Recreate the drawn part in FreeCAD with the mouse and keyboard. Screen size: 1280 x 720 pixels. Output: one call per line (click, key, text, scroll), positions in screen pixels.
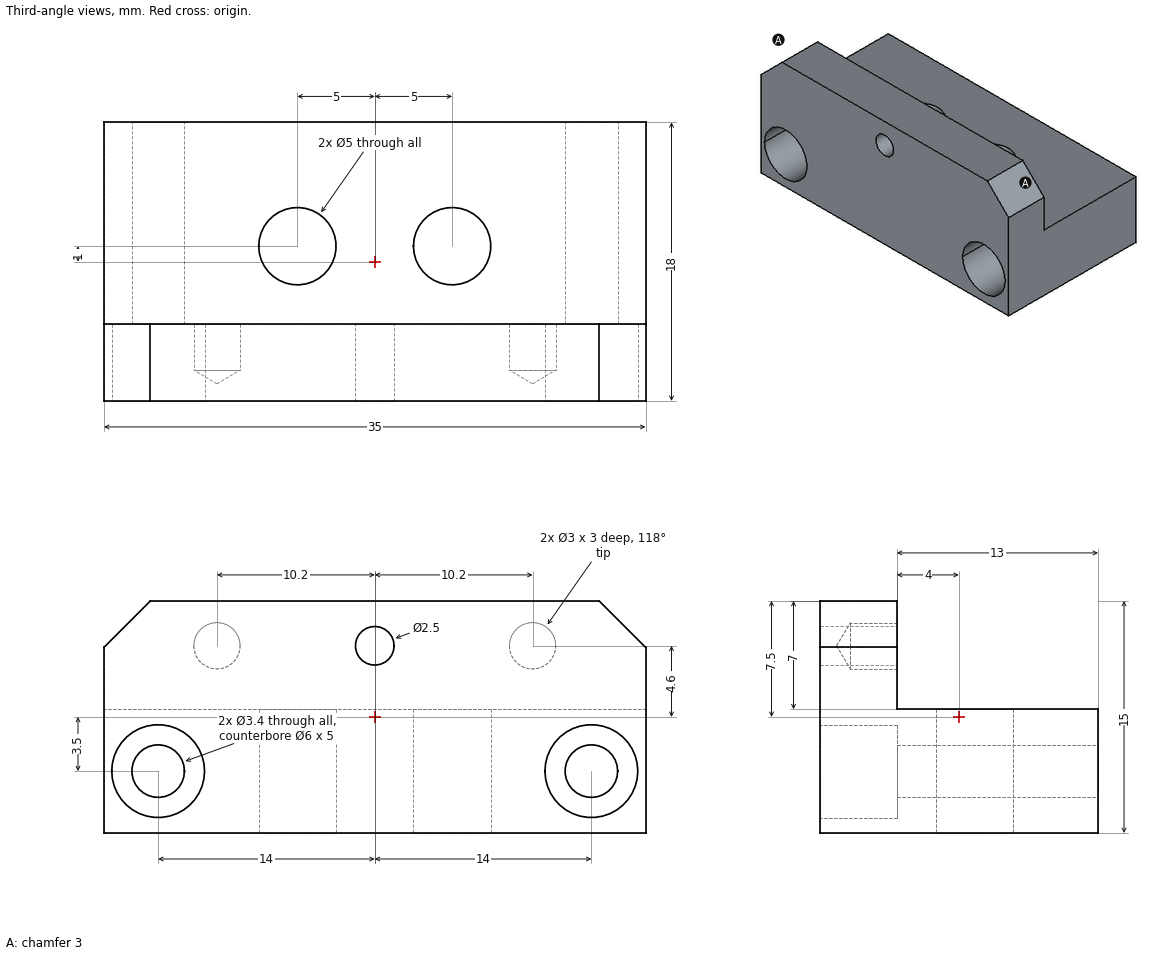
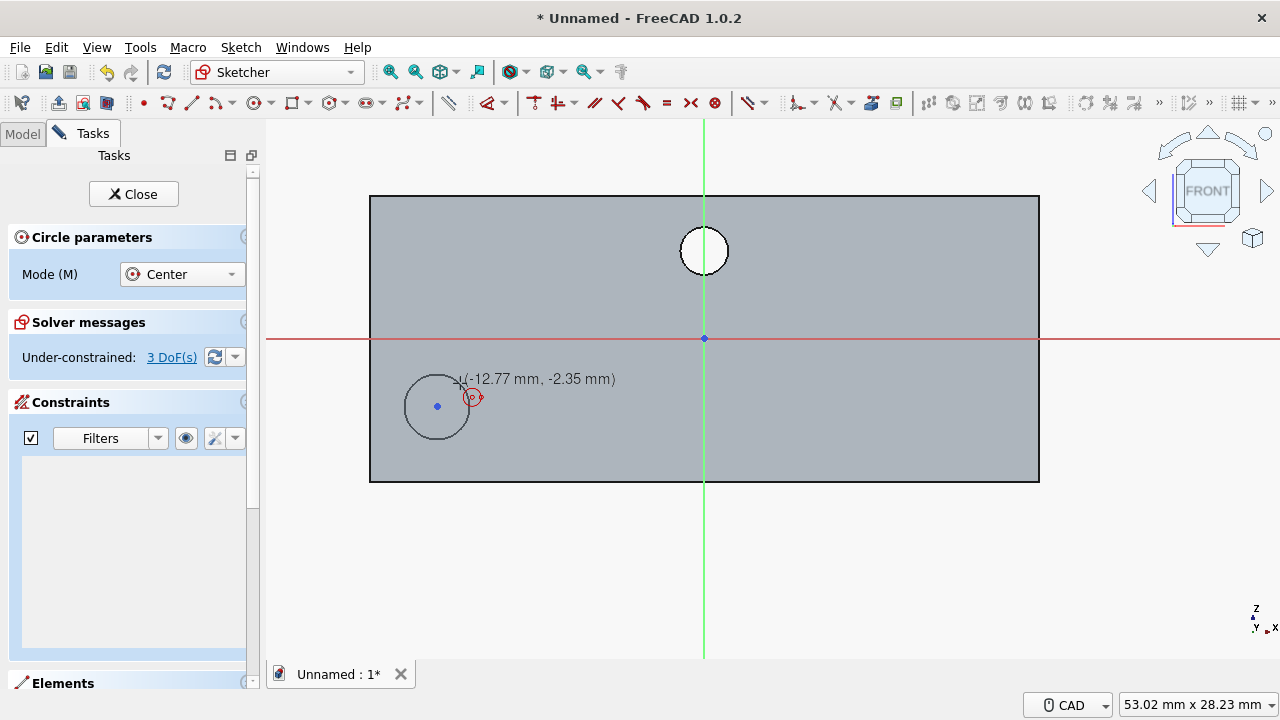
click(972, 406)
click(995, 383)
key(Escape)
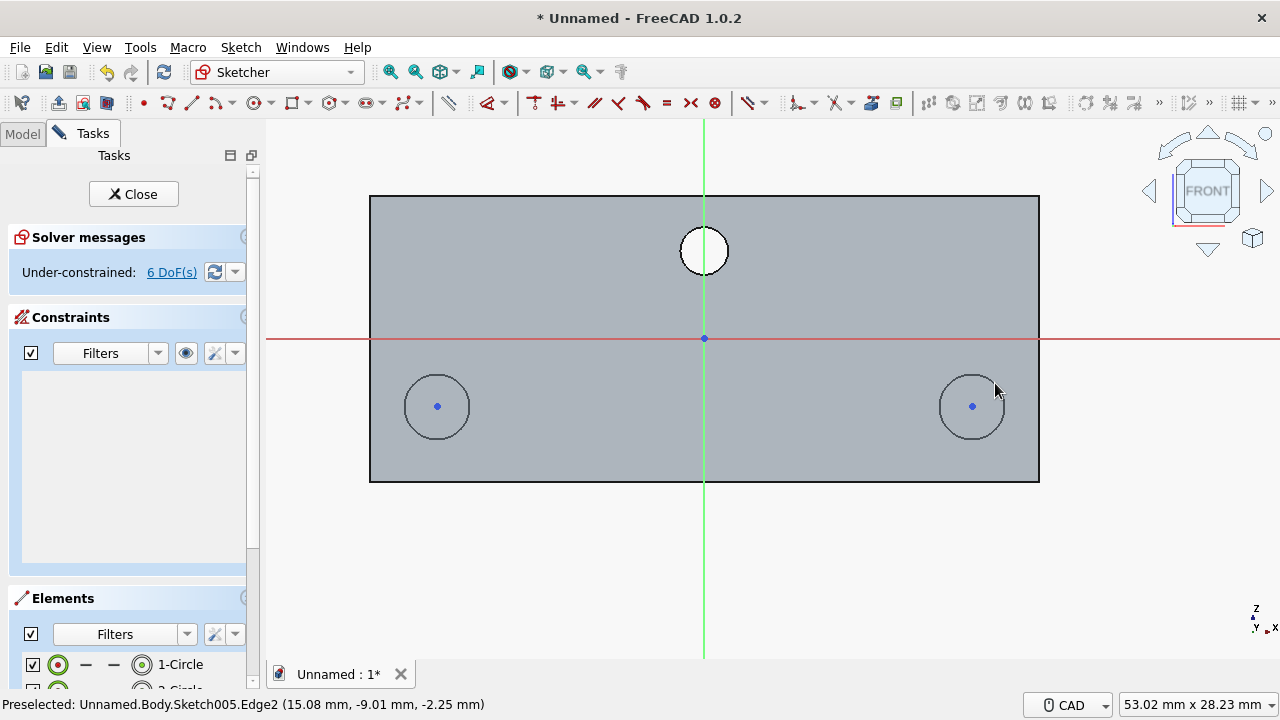
click(460, 384)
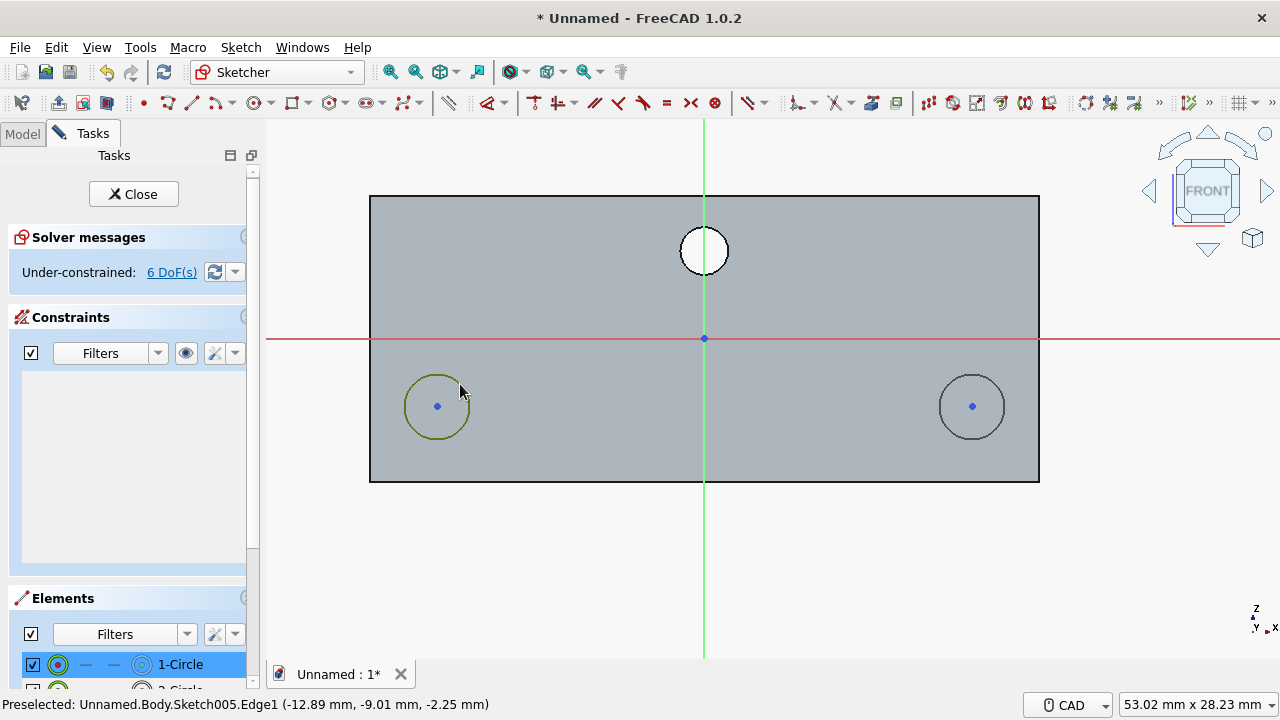
click(995, 384)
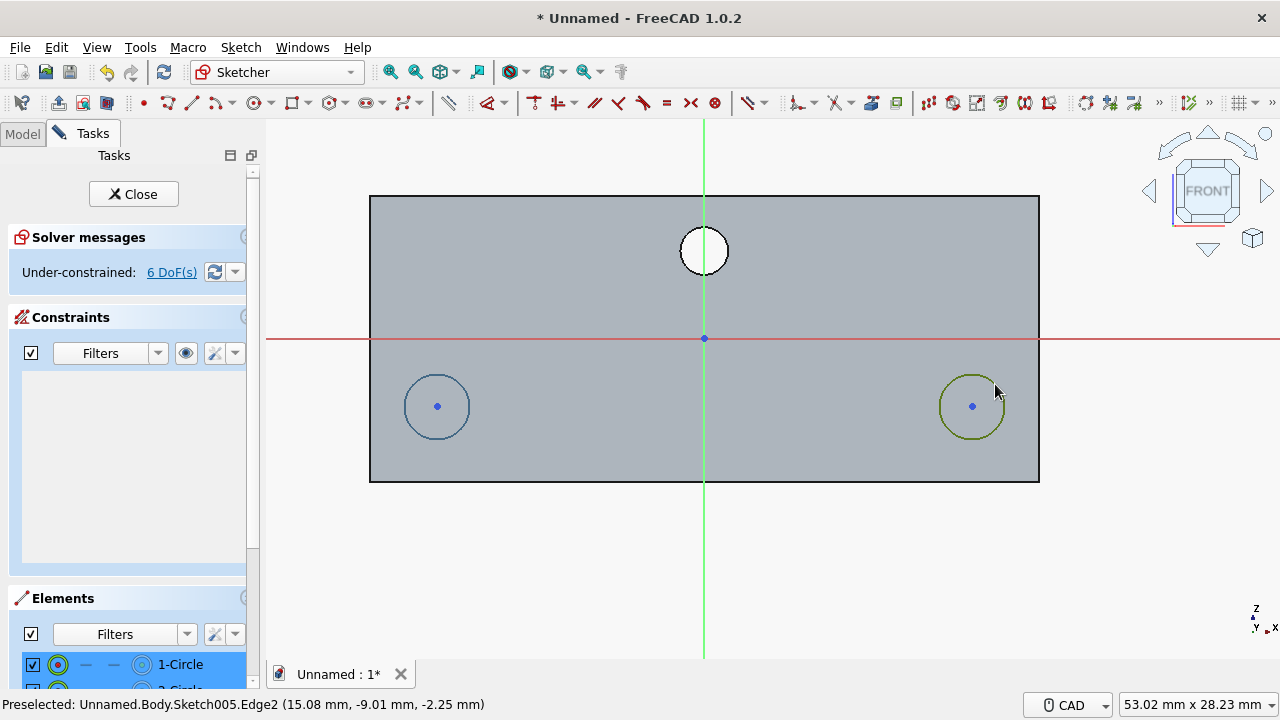
key(e)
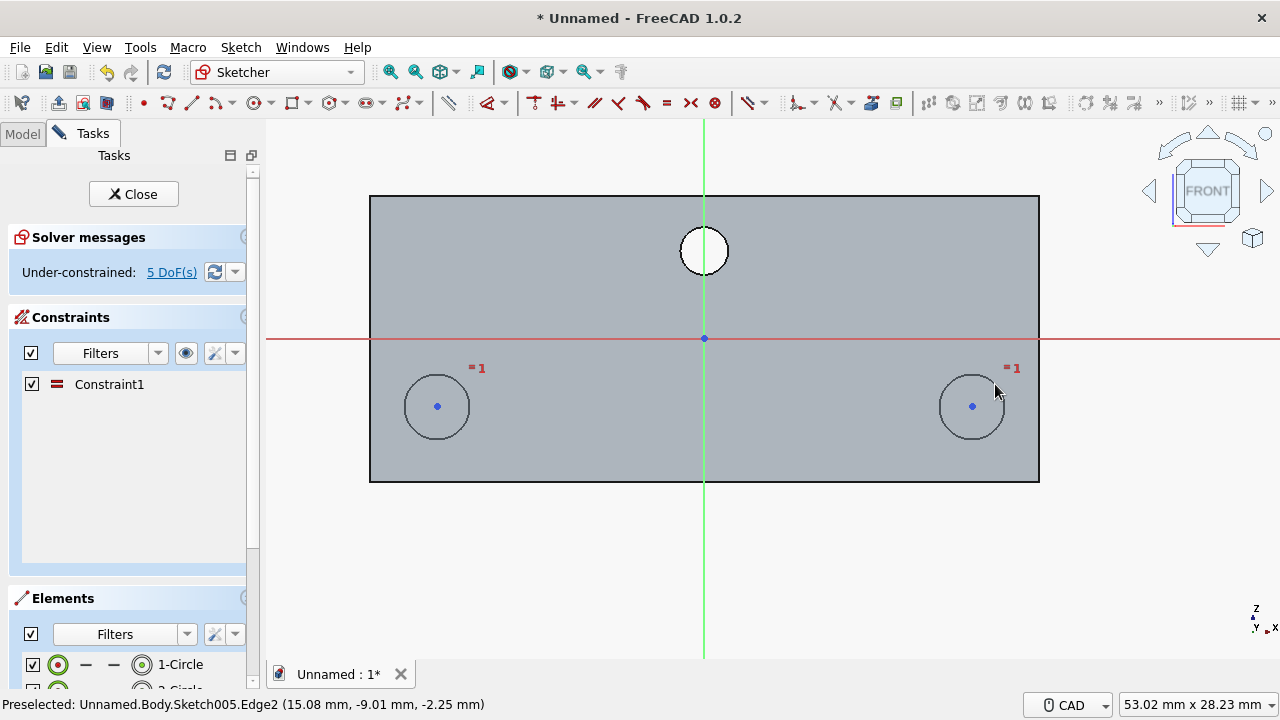
click(437, 407)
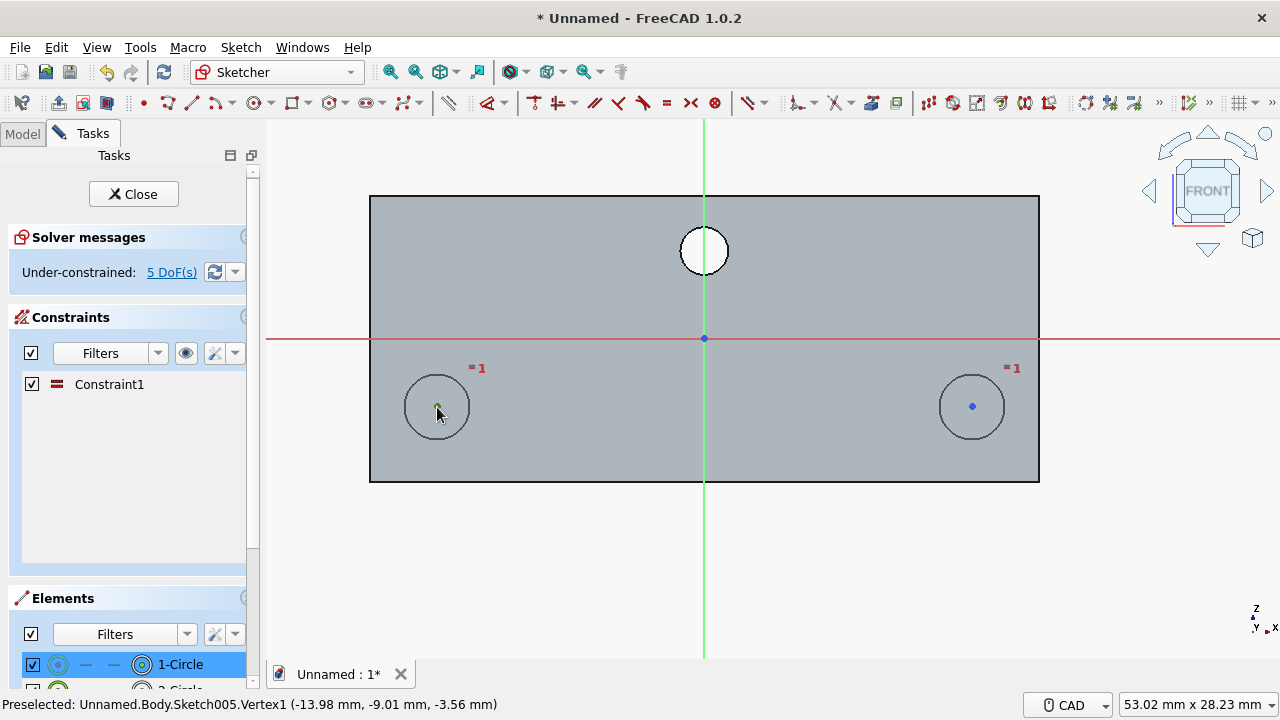
click(972, 407)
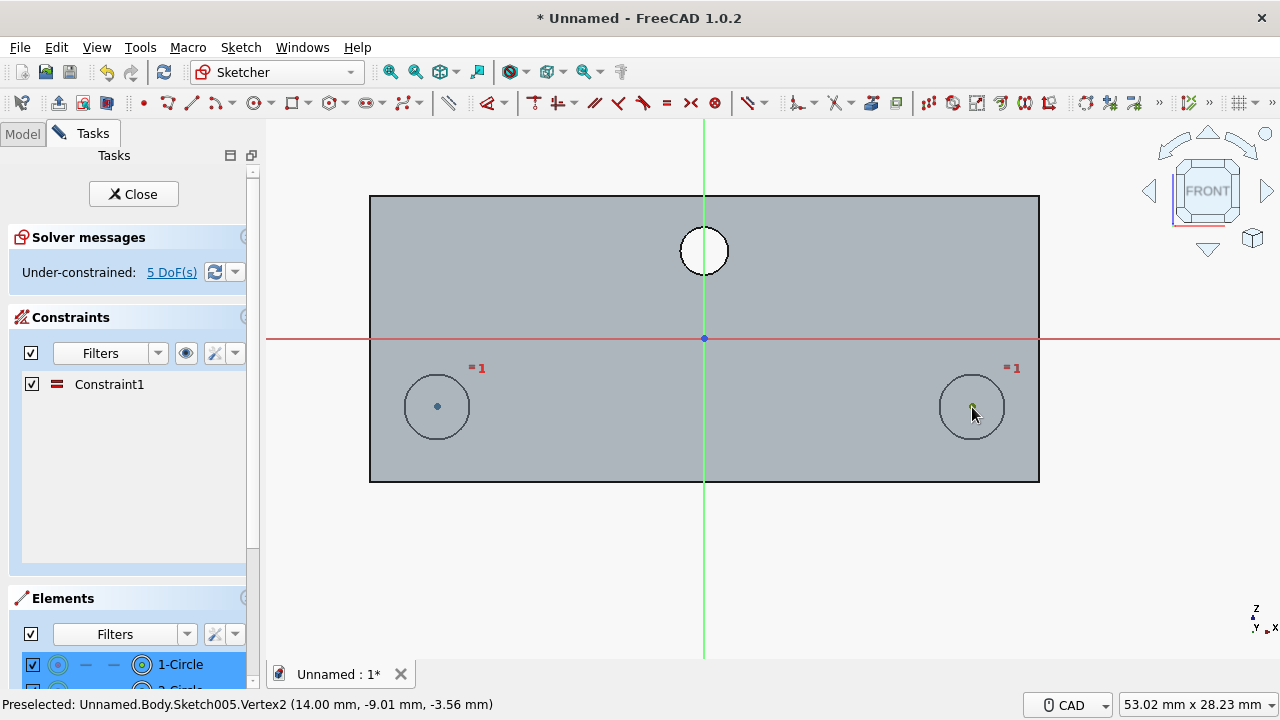
key(h)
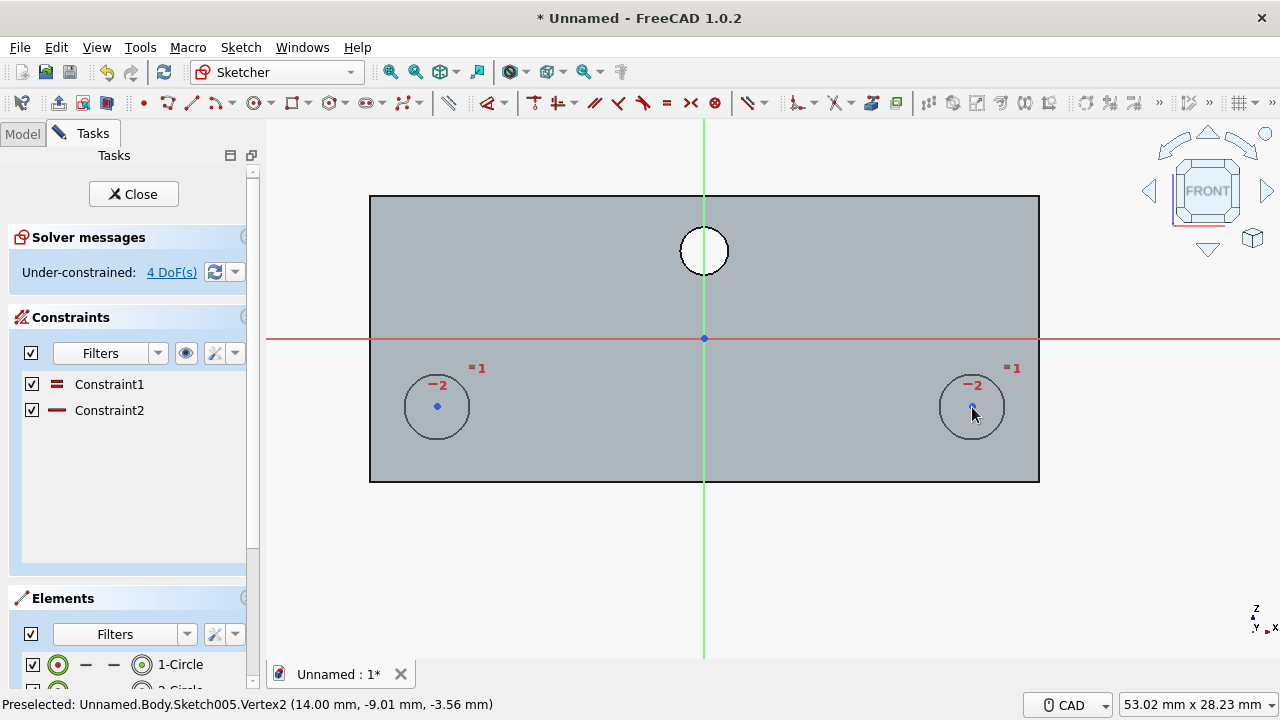
key(d)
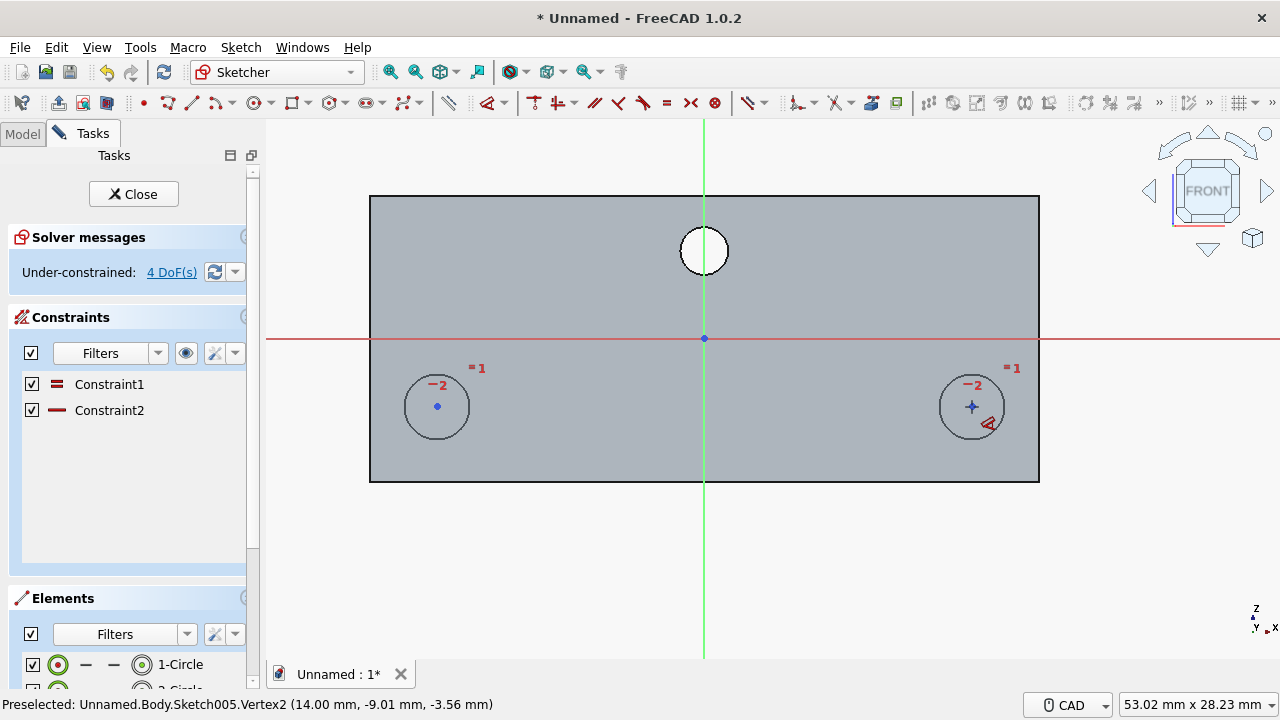
click(460, 384)
click(483, 361)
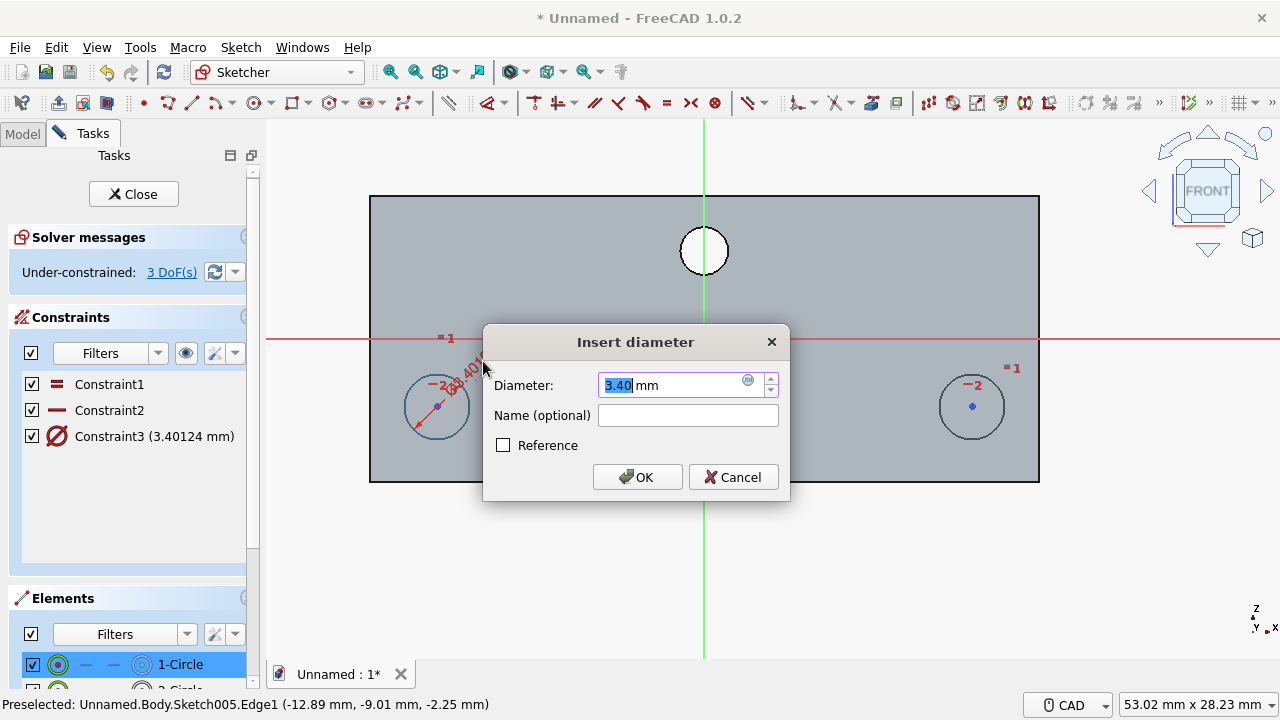
text(3.4)
key(Return)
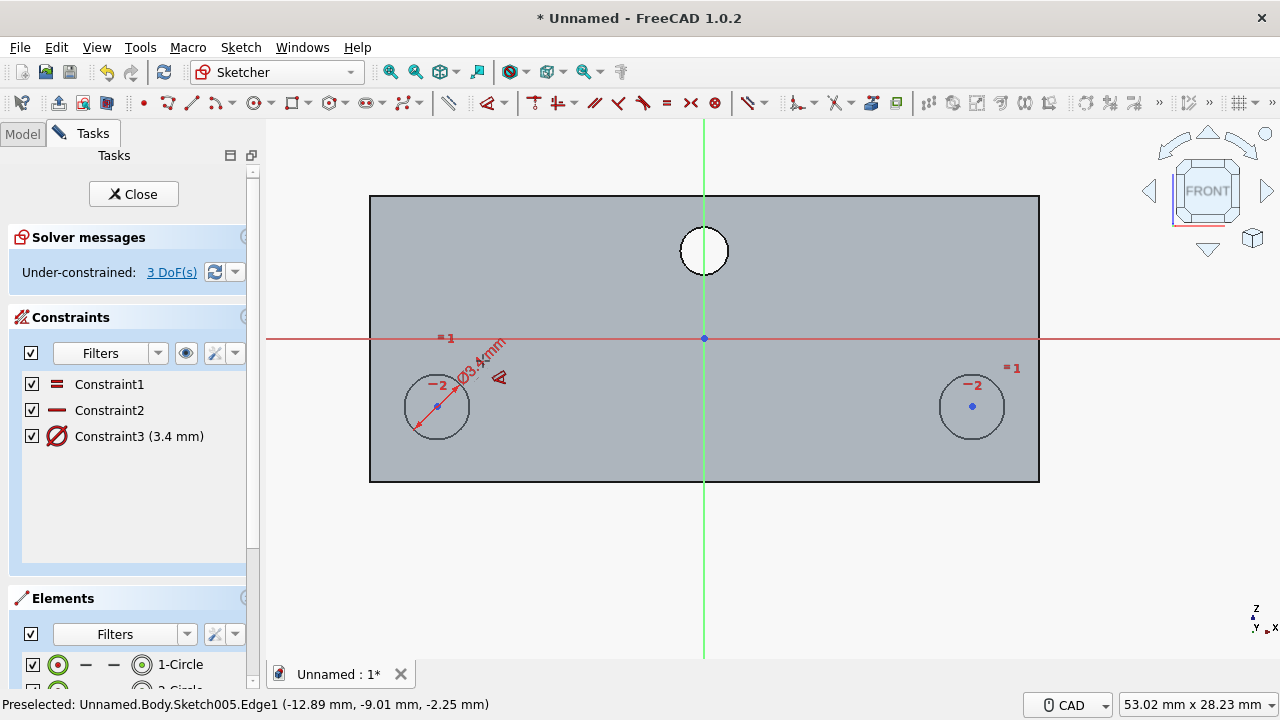
click(437, 407)
click(571, 305)